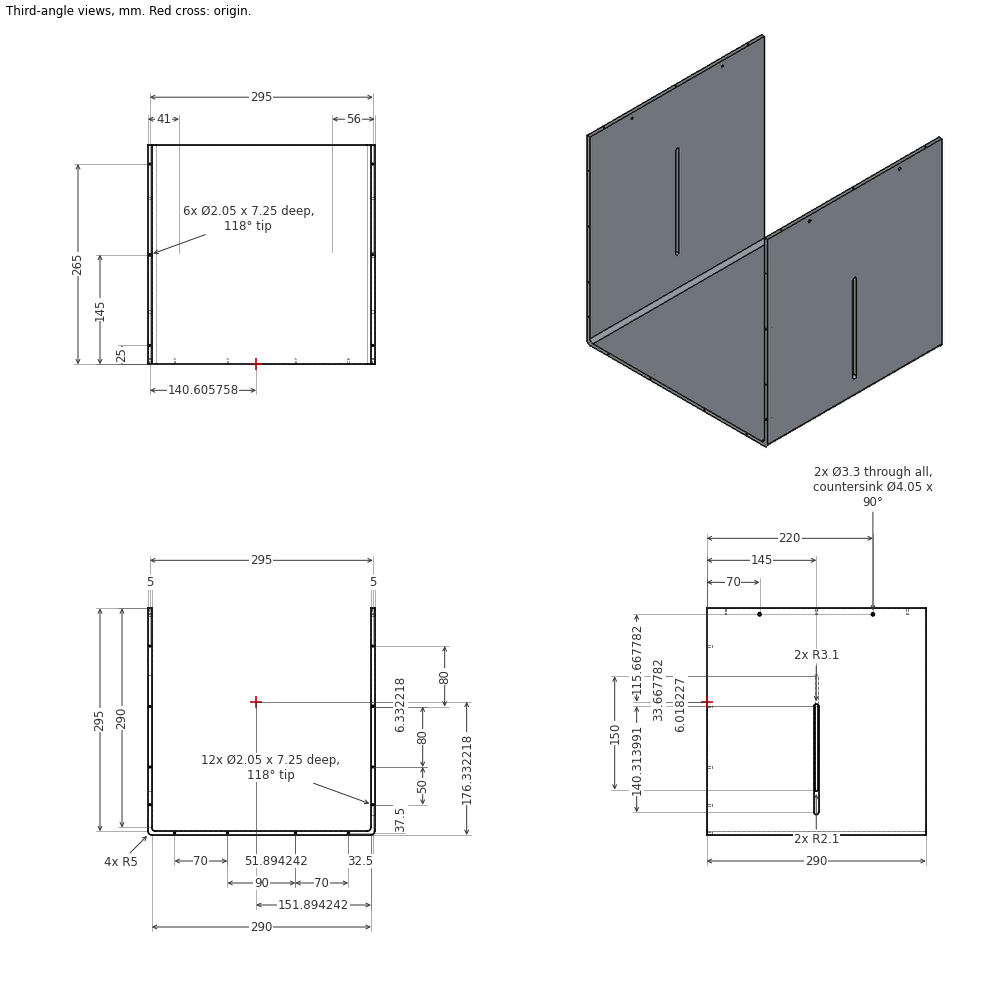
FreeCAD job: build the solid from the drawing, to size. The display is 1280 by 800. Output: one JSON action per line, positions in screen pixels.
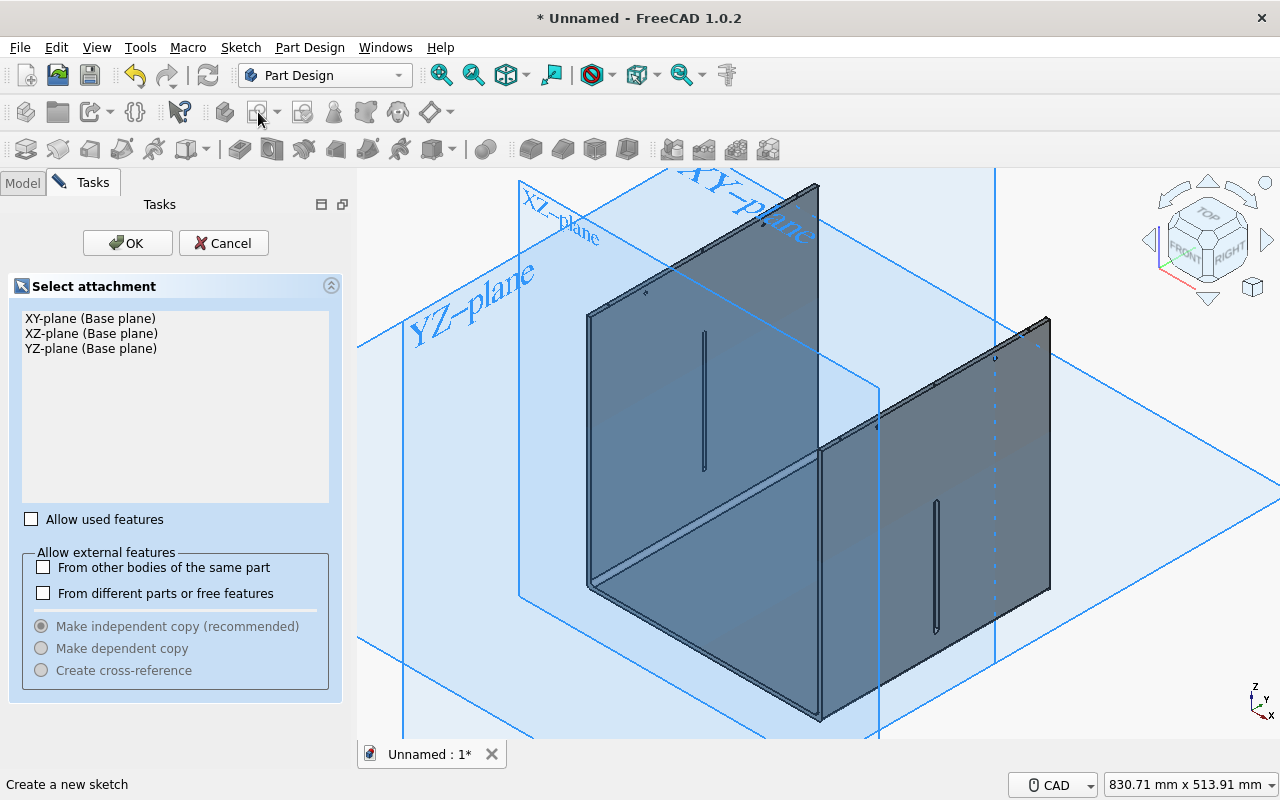
{"action": "left_click", "coordinate": [82, 334]}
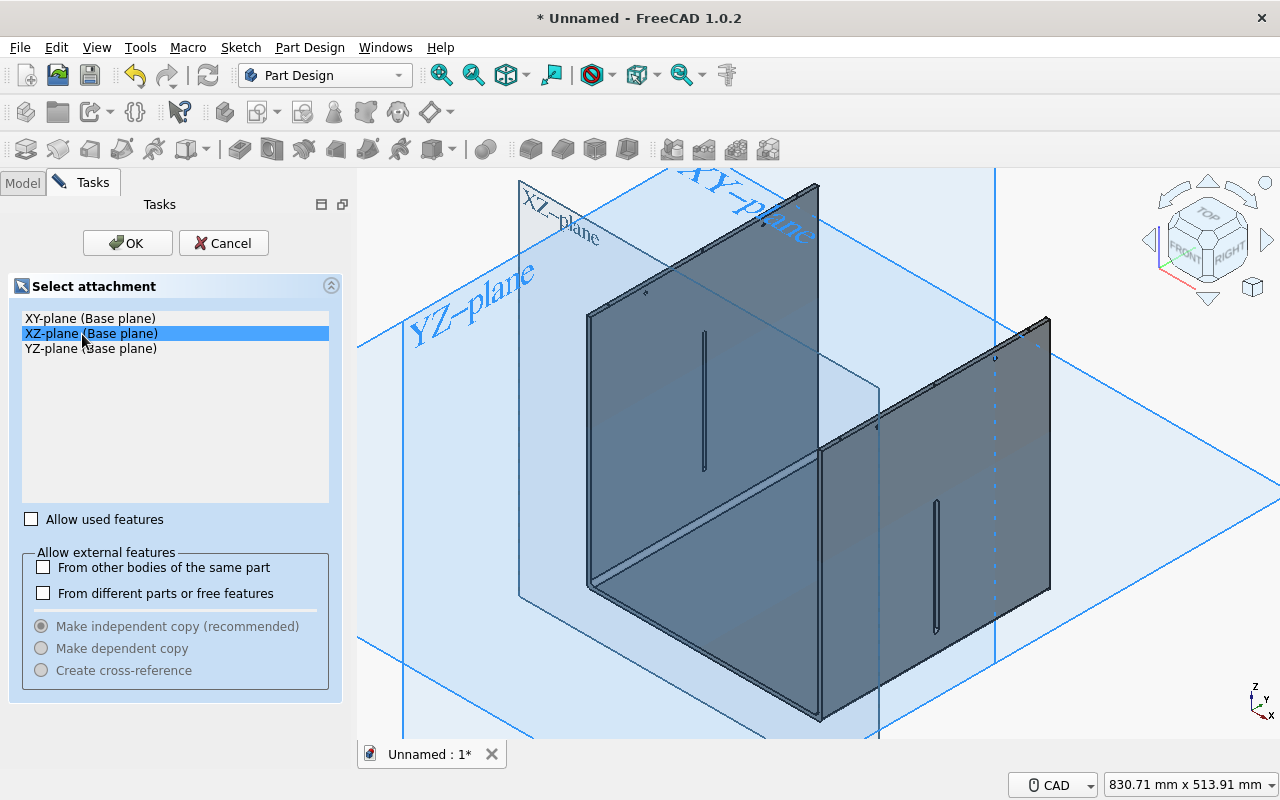
{"action": "left_click", "coordinate": [128, 243]}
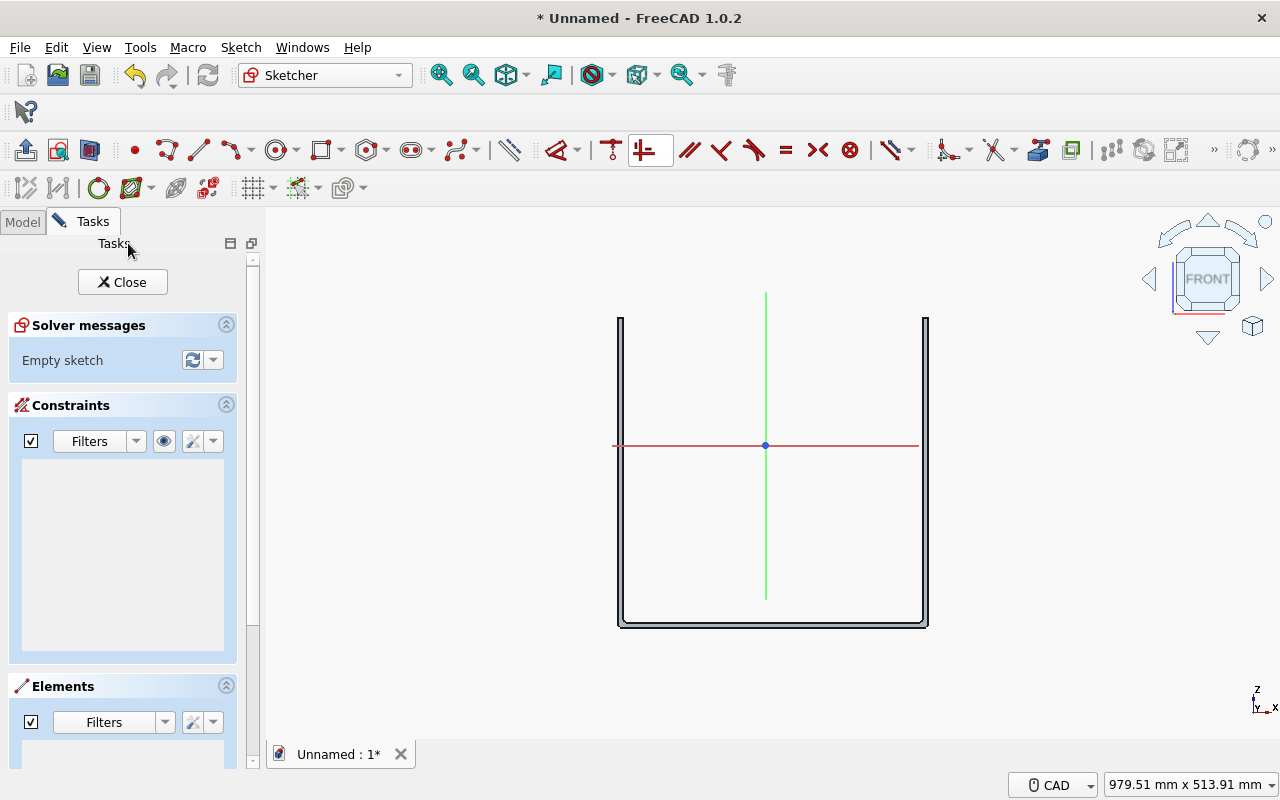
{"action": "left_click", "coordinate": [276, 150]}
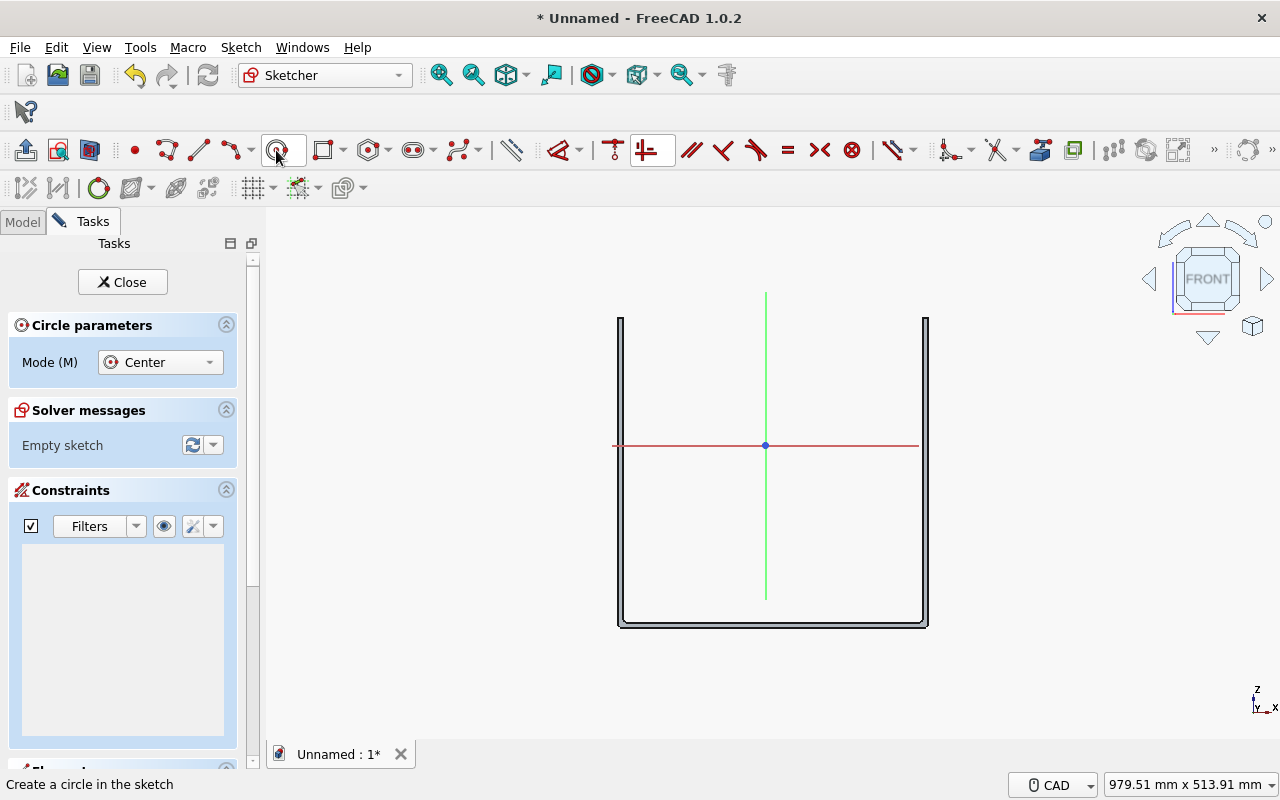
{"action": "scroll", "coordinate": [926, 587], "scroll_direction": "up", "scroll_amount": 16}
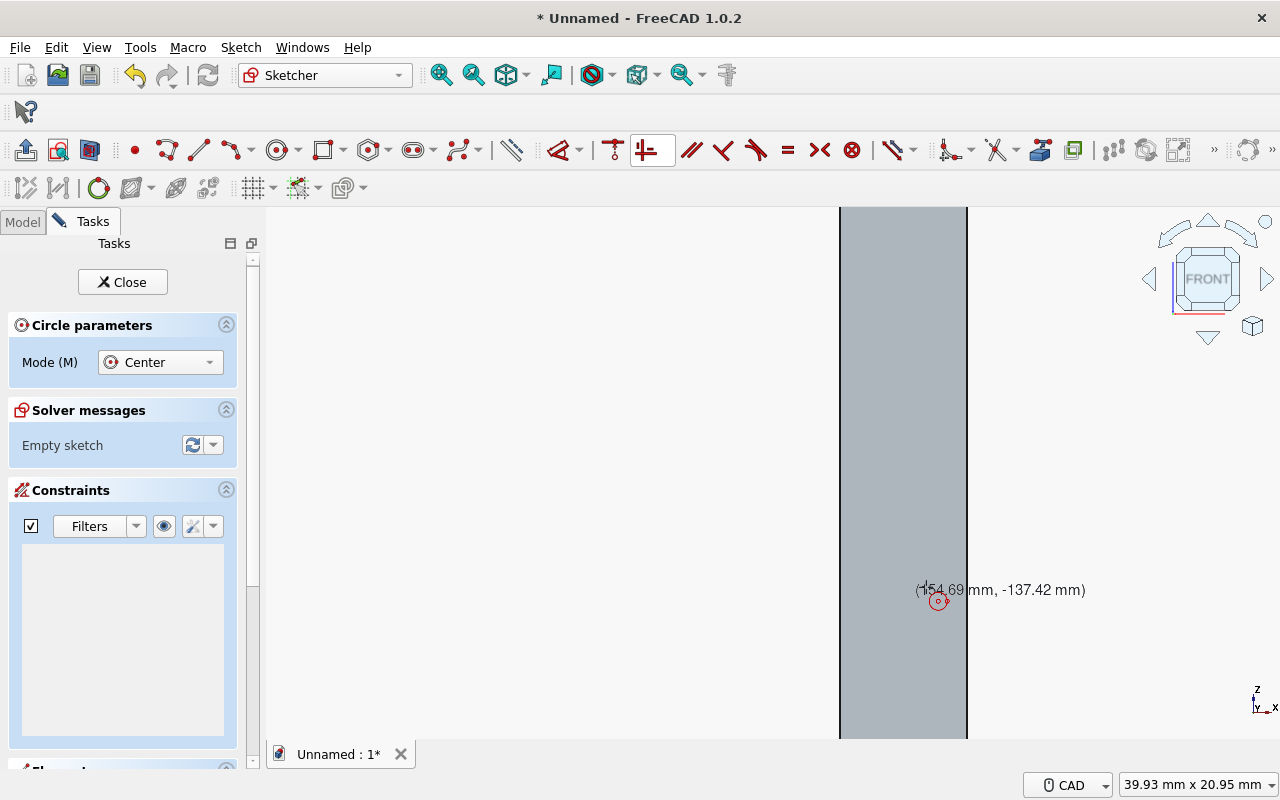
{"action": "scroll", "coordinate": [890, 583], "scroll_direction": "down", "scroll_amount": 15}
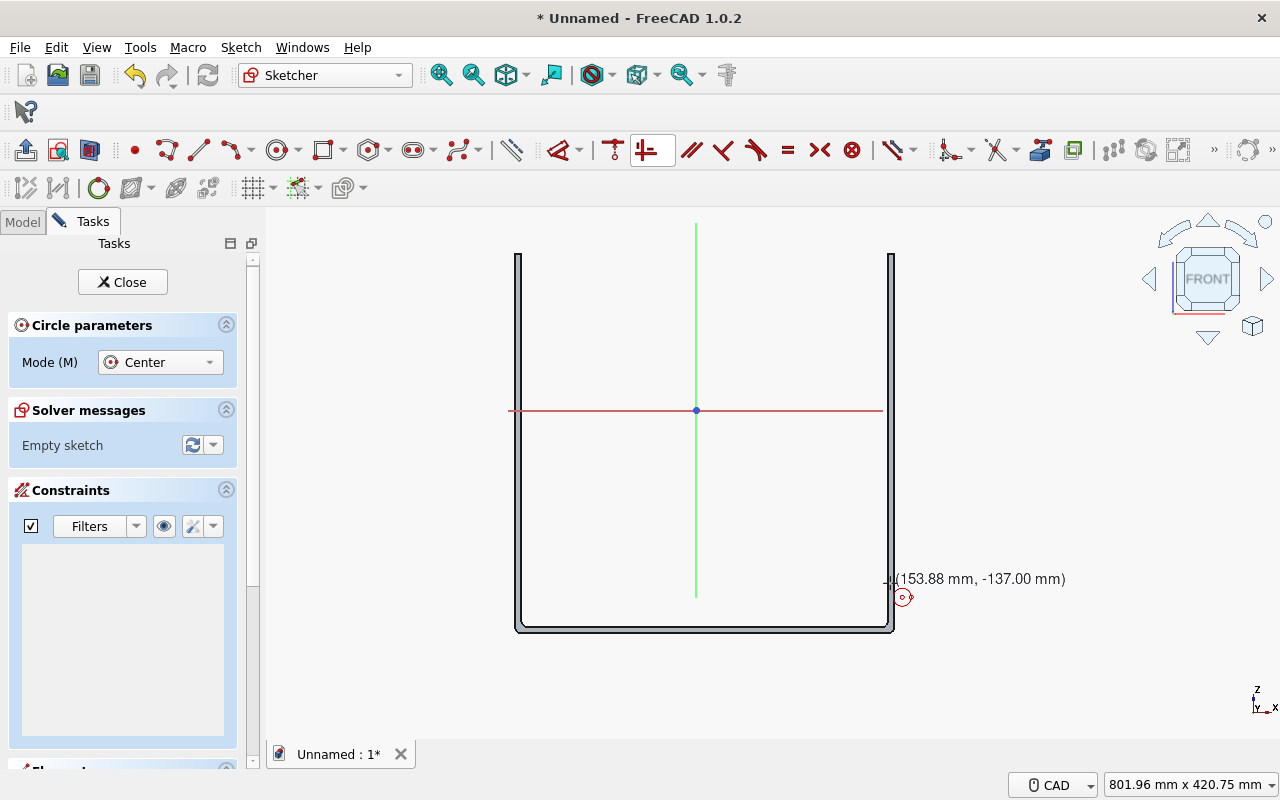
{"action": "left_click", "coordinate": [891, 583]}
{"action": "mouse_move", "coordinate": [892, 582]}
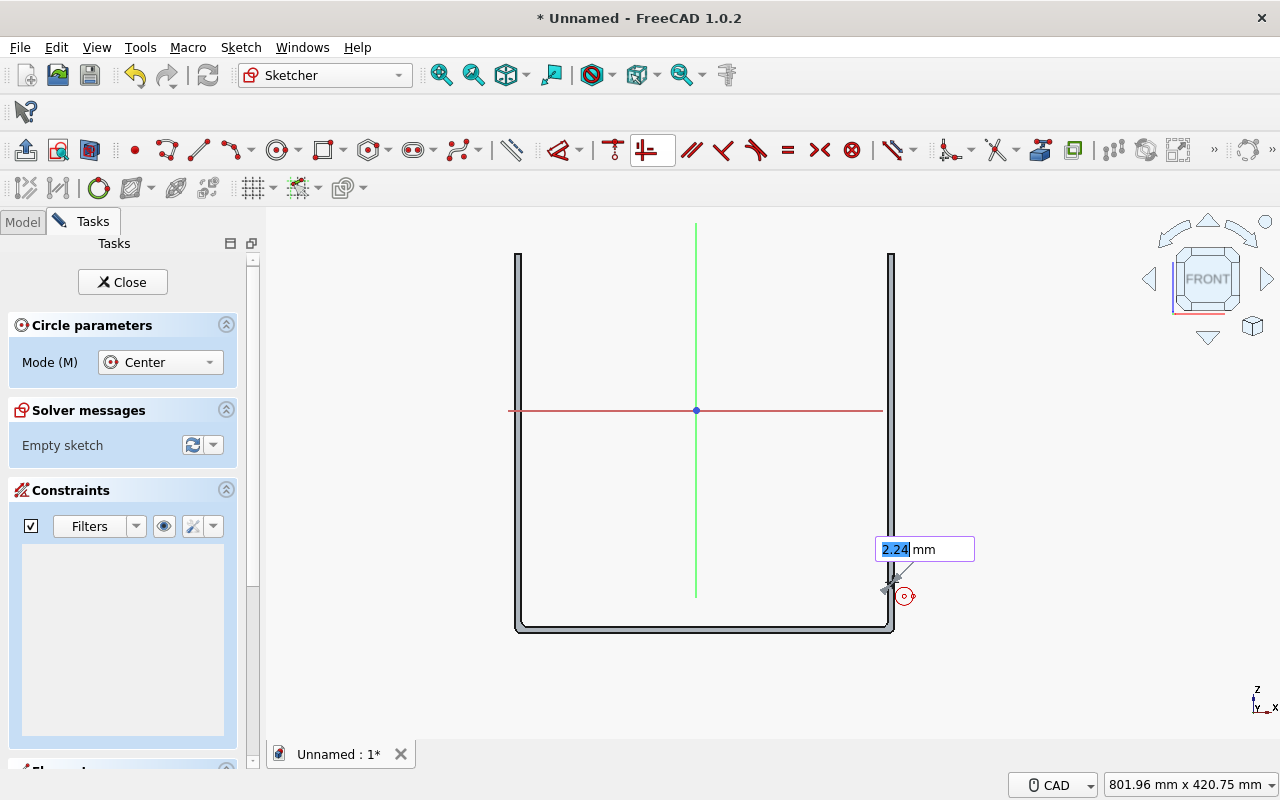
{"action": "type", "text": "2.05"}
{"action": "key", "text": "Return"}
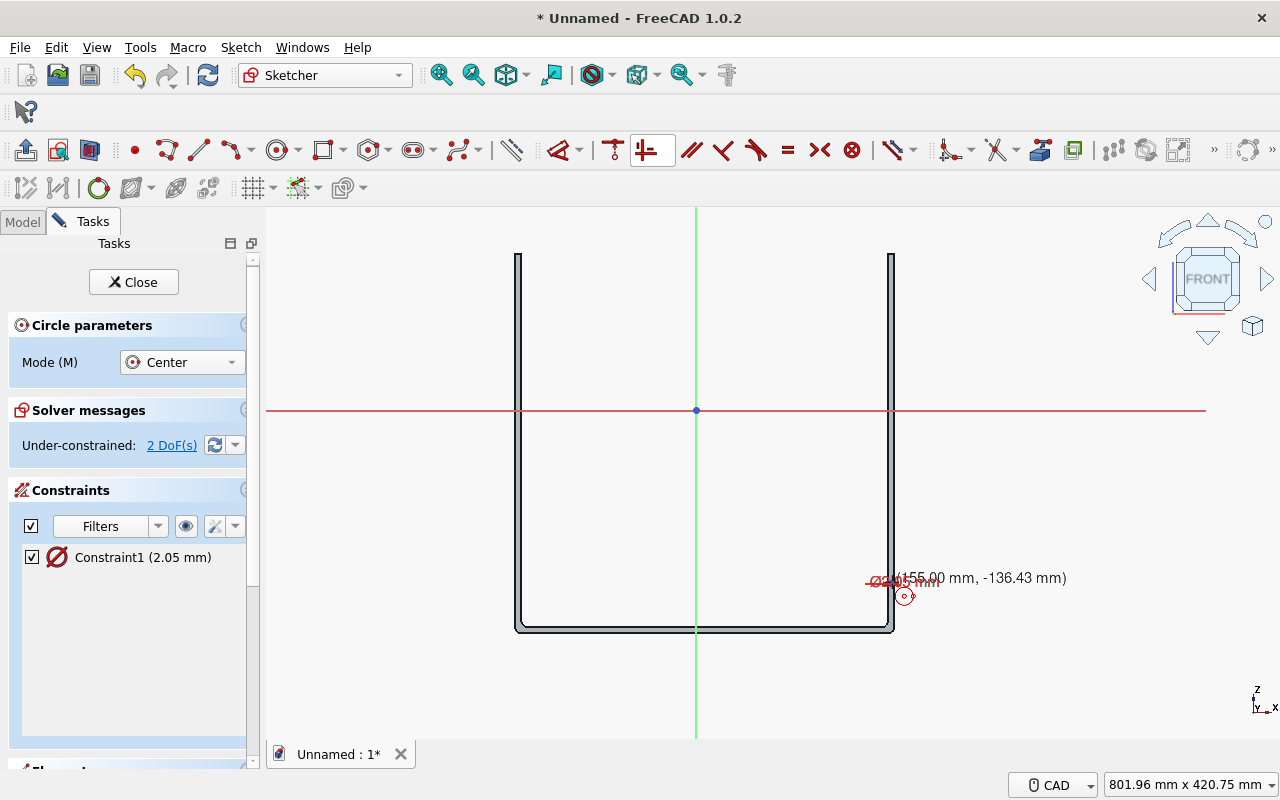
{"action": "scroll", "coordinate": [891, 520], "scroll_direction": "up", "scroll_amount": 15}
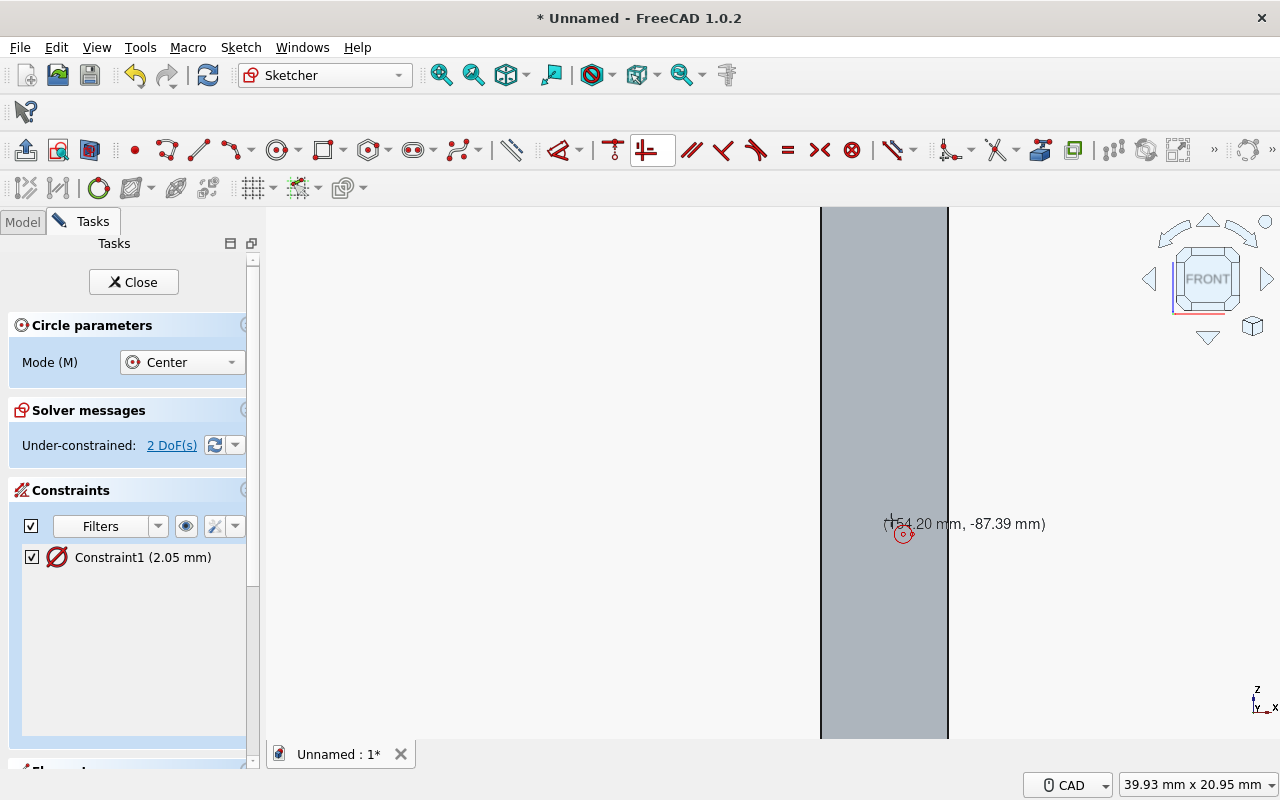
{"action": "scroll", "coordinate": [891, 520], "scroll_direction": "down", "scroll_amount": 15}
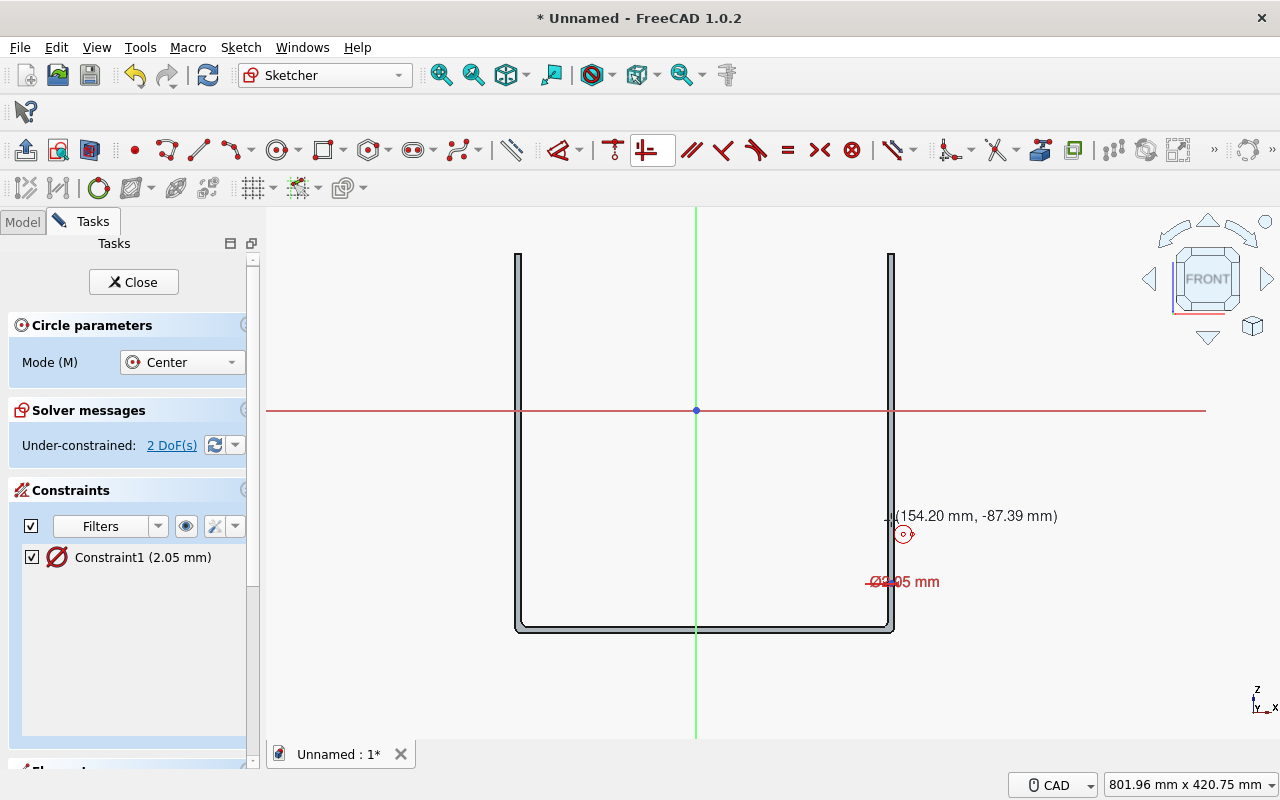
{"action": "left_click", "coordinate": [891, 520]}
{"action": "mouse_move", "coordinate": [892, 519]}